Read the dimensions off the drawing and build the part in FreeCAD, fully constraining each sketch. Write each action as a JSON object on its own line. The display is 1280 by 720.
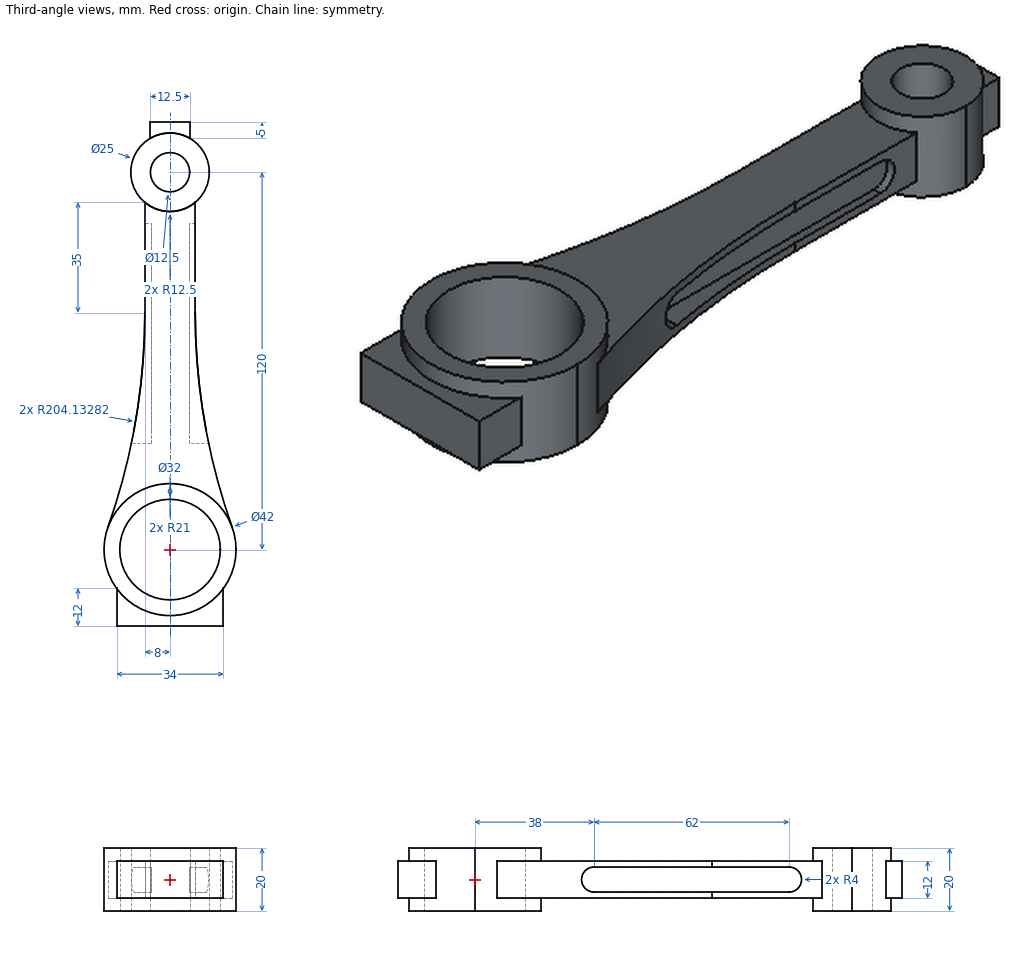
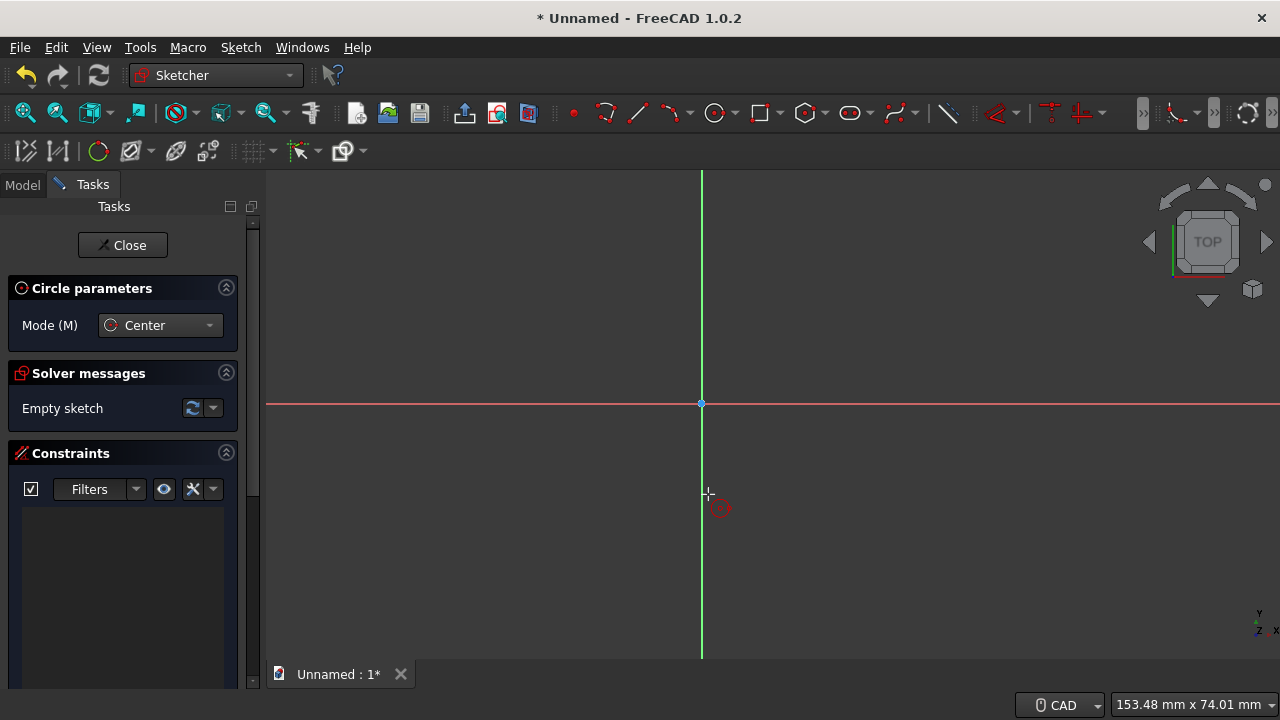
{"action": "left_click", "coordinate": [702, 404]}
{"action": "left_click", "coordinate": [800, 306]}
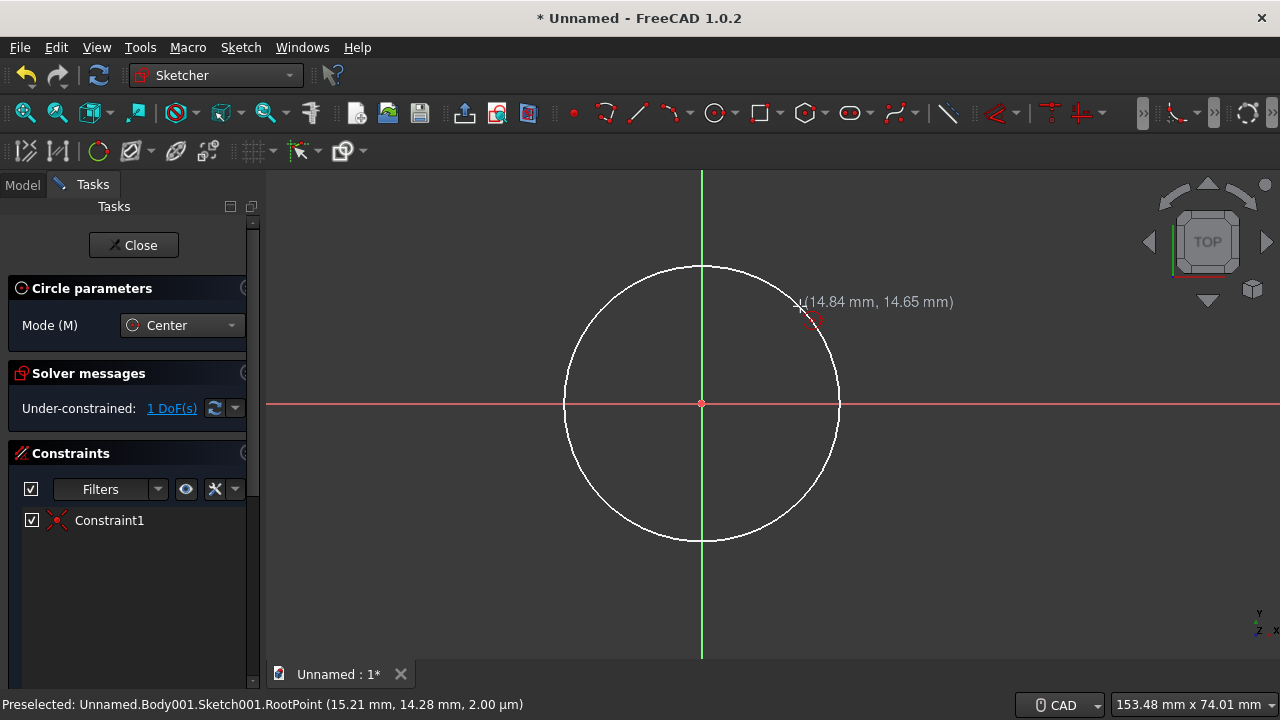
{"action": "left_click", "coordinate": [702, 404]}
{"action": "left_click", "coordinate": [777, 329]}
{"action": "key", "text": "Escape"}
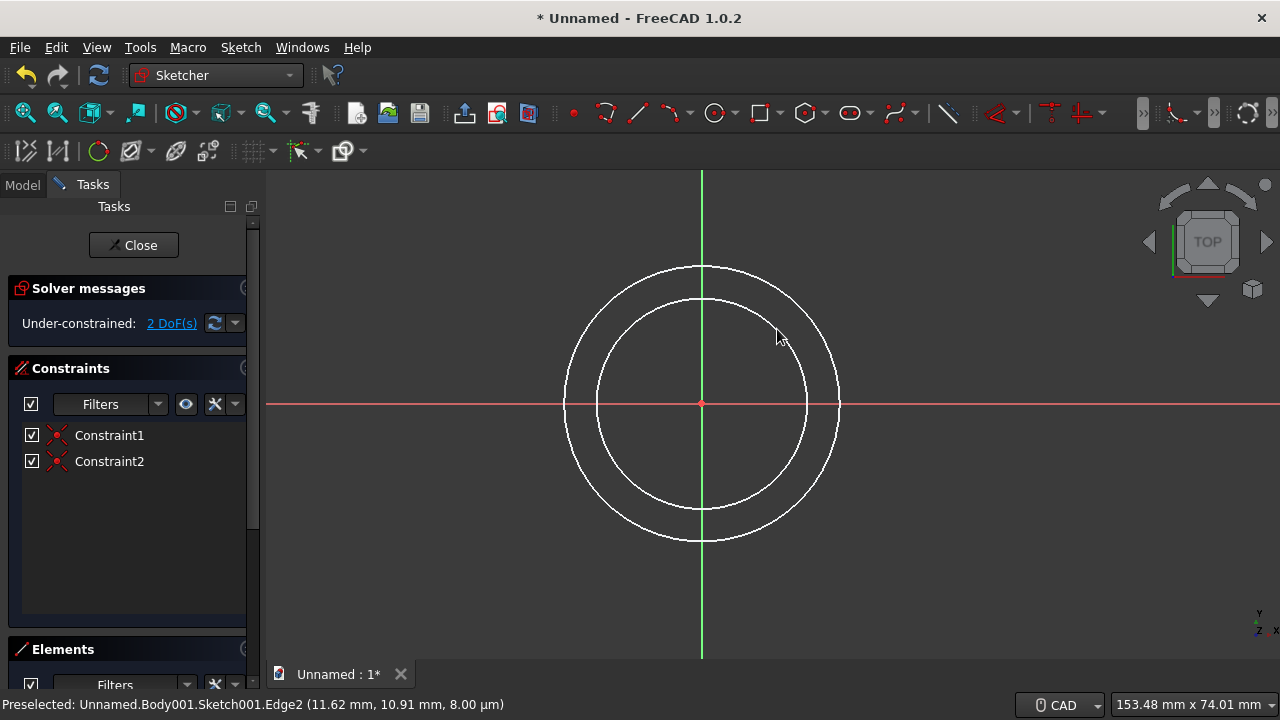
{"action": "key", "text": "d"}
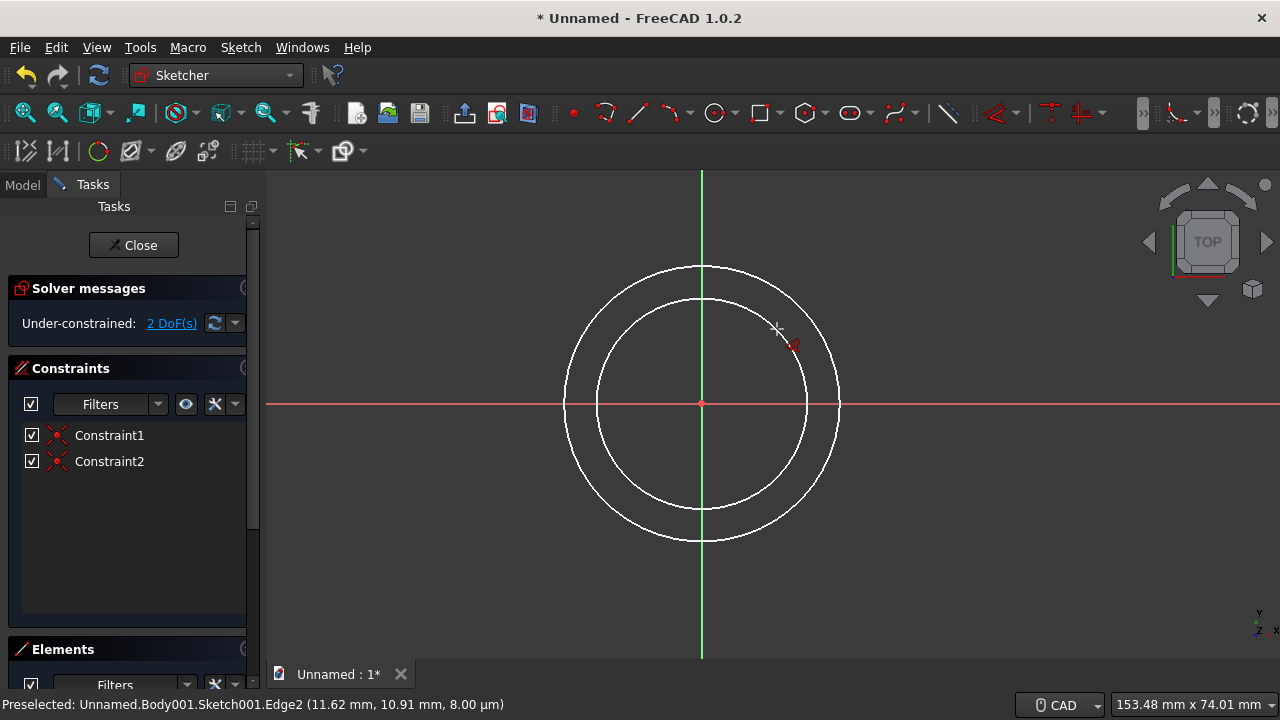
{"action": "left_click", "coordinate": [799, 306]}
{"action": "left_click", "coordinate": [822, 283]}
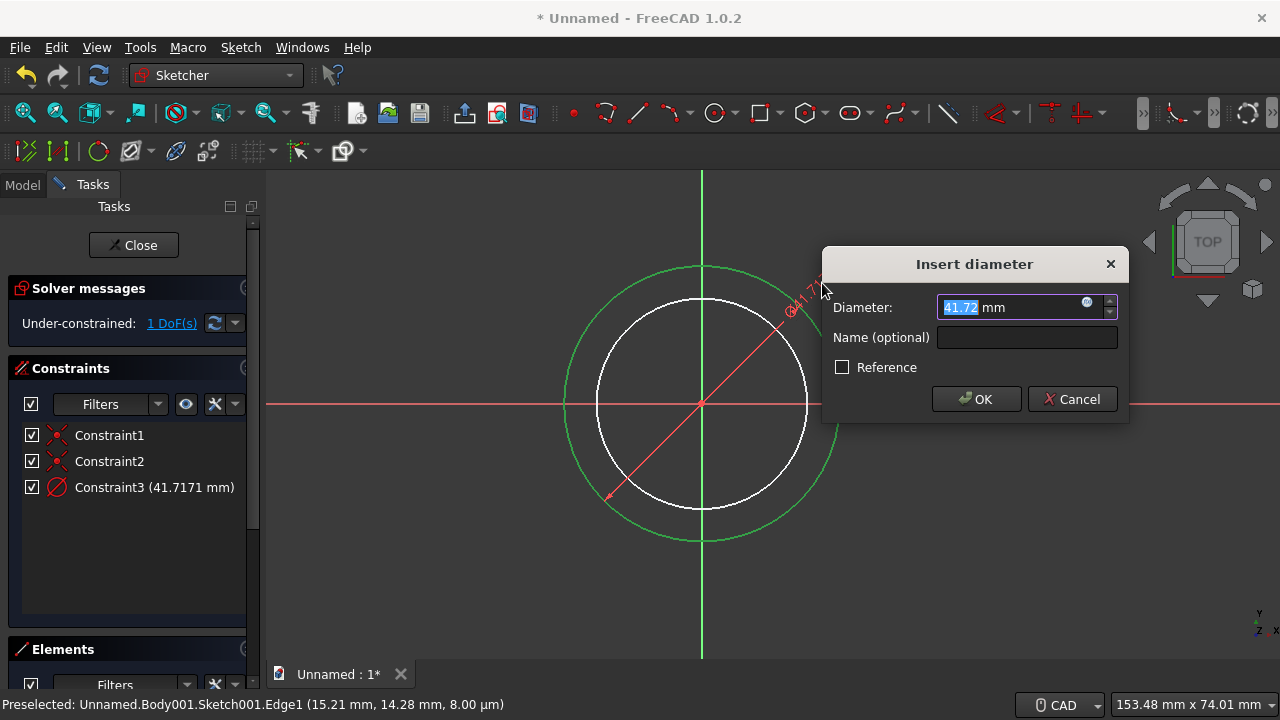
{"action": "type", "text": "42"}
{"action": "key", "text": "Return"}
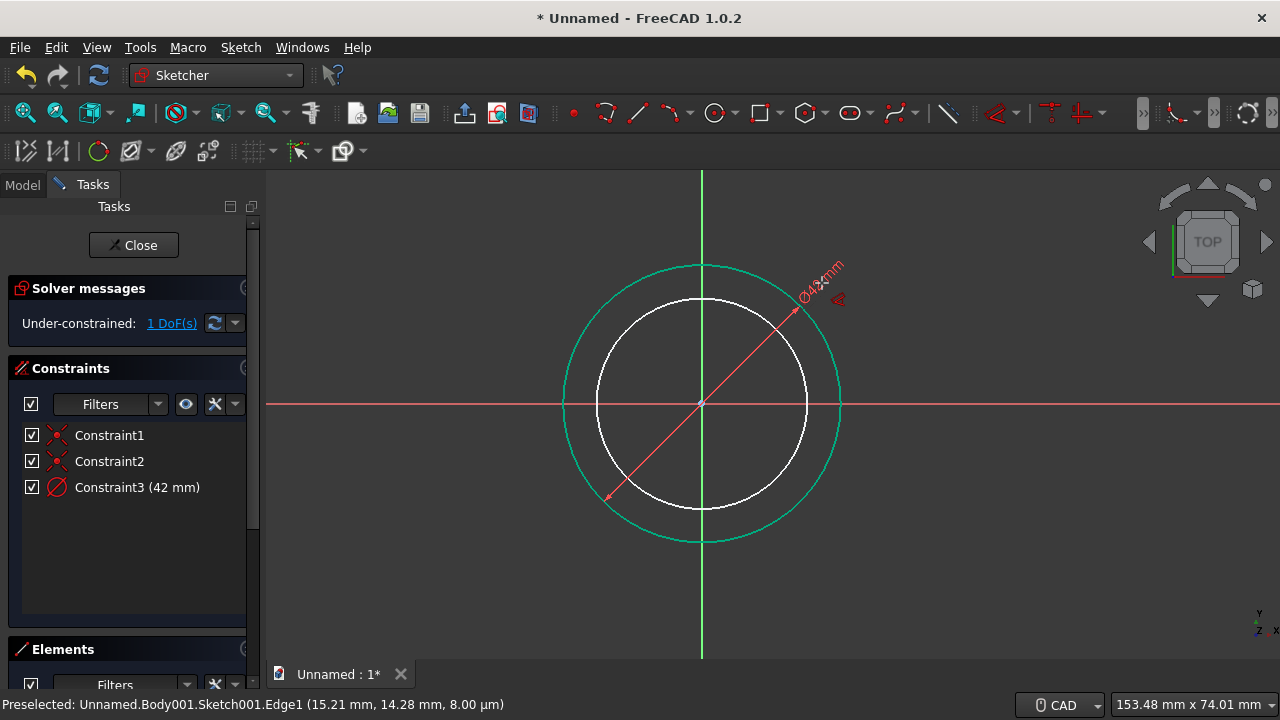
{"action": "left_click", "coordinate": [776, 329]}
{"action": "left_click", "coordinate": [855, 358]}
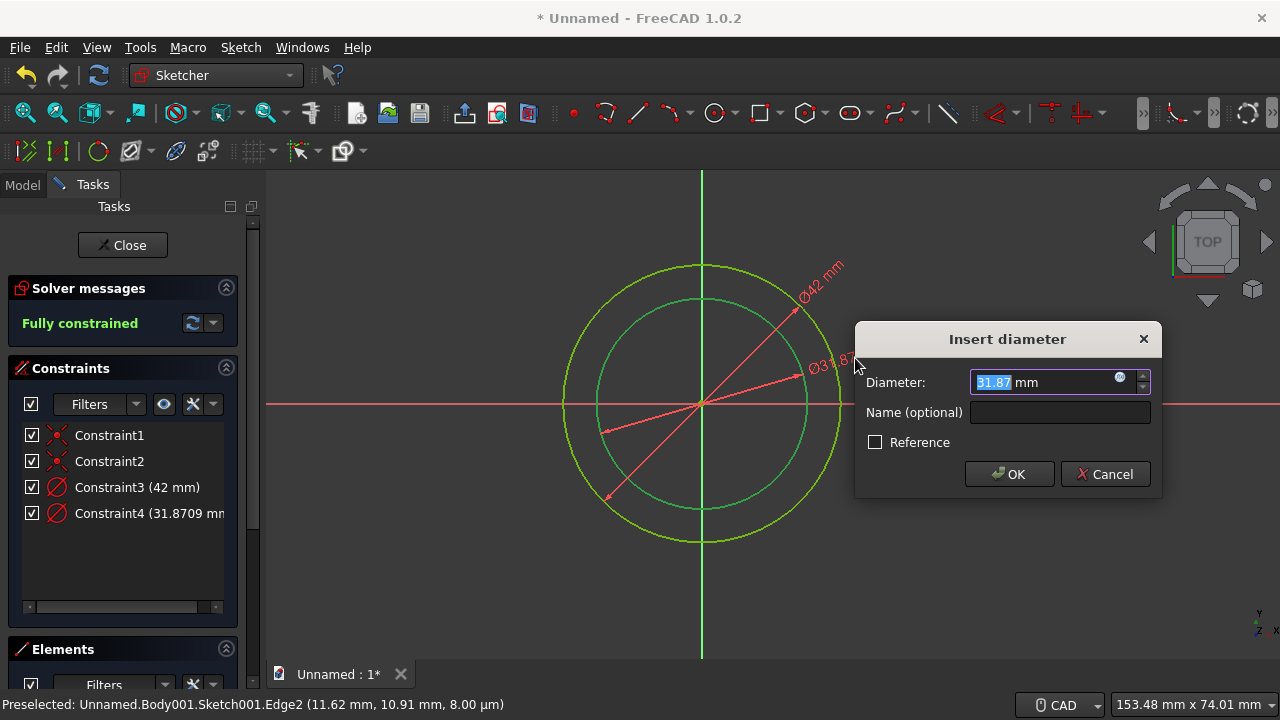
{"action": "type", "text": "32"}
{"action": "key", "text": "Return"}
{"action": "key", "text": "Escape"}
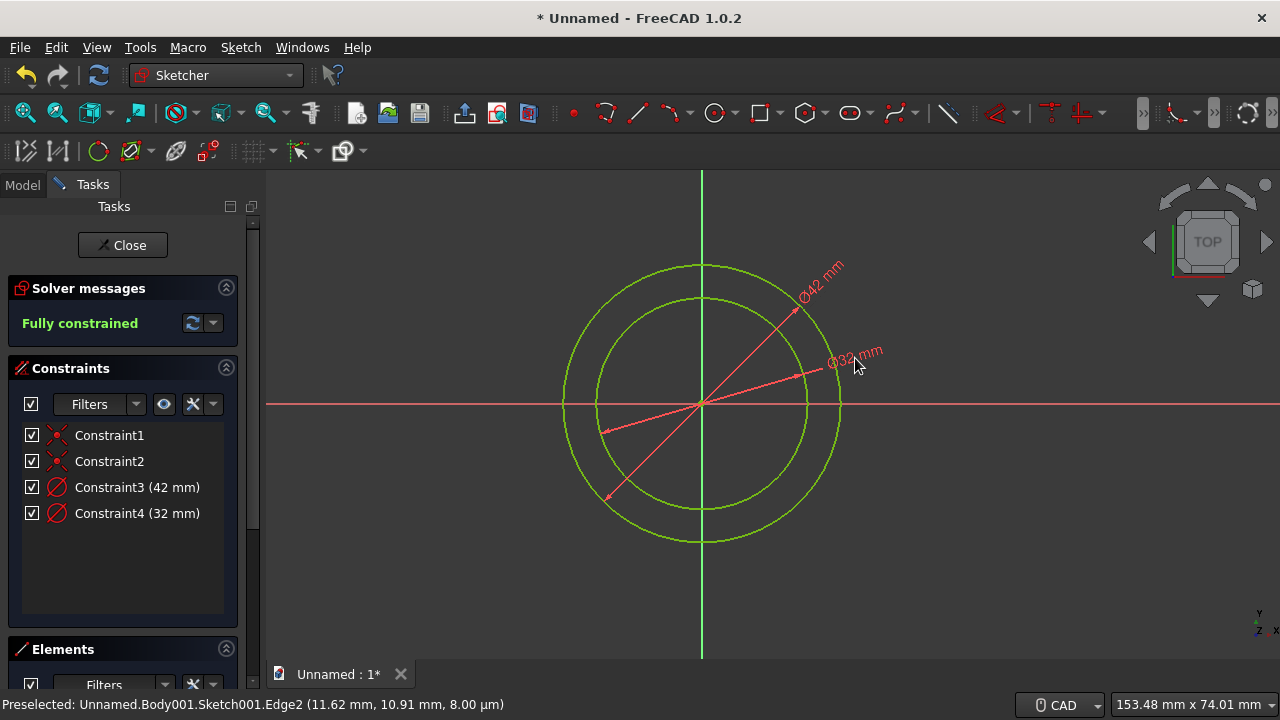
{"action": "left_click", "coordinate": [123, 245]}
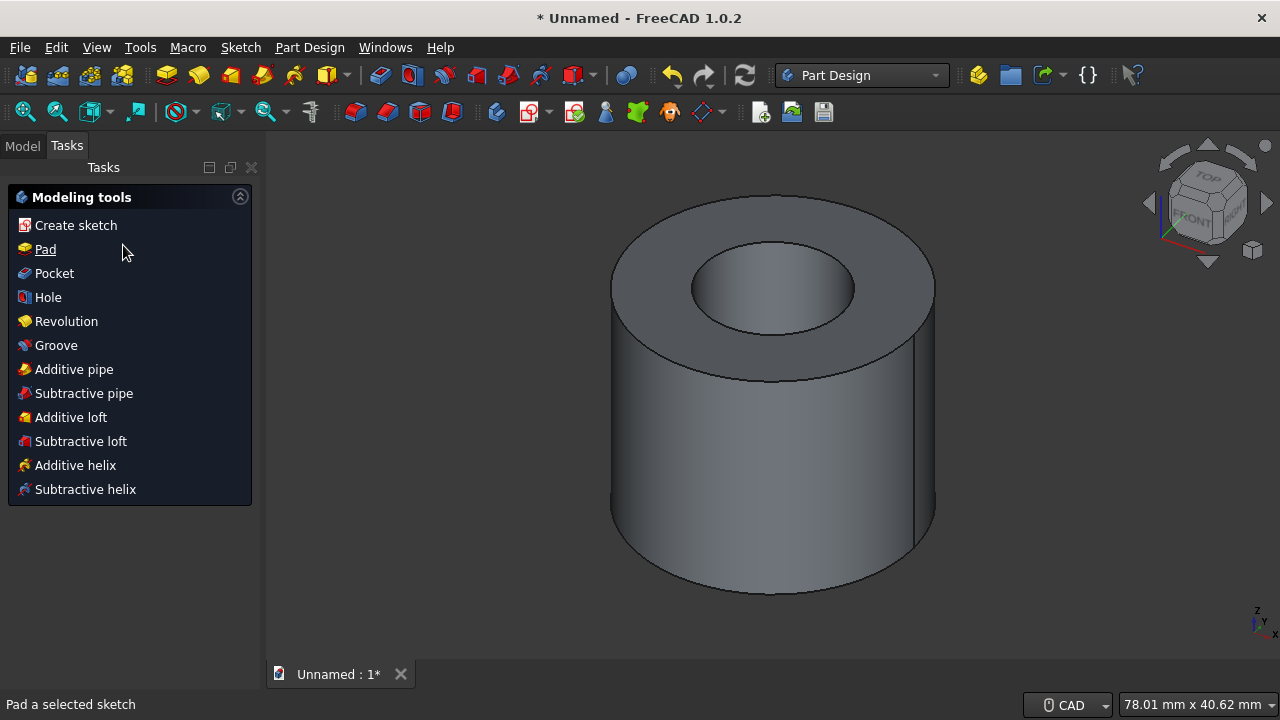
{"action": "left_click", "coordinate": [168, 76]}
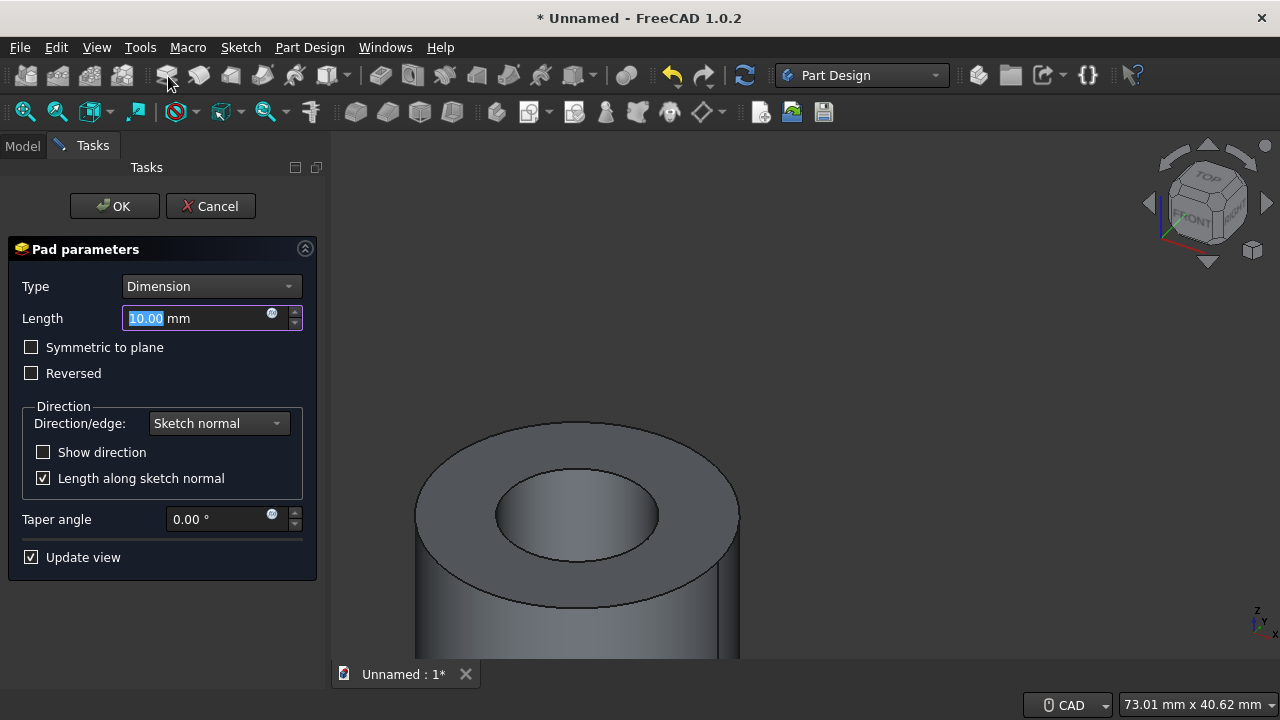
{"action": "type", "text": "20"}
{"action": "key", "text": "Tab"}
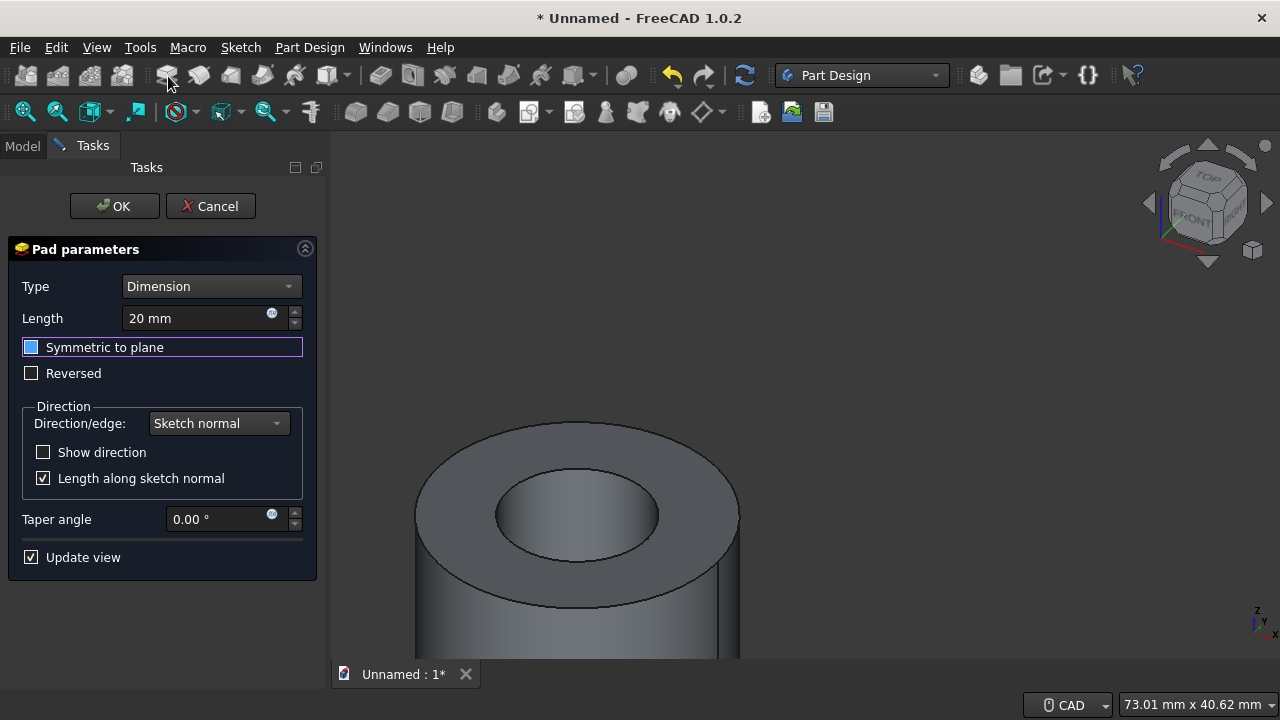
{"action": "left_click", "coordinate": [30, 347]}